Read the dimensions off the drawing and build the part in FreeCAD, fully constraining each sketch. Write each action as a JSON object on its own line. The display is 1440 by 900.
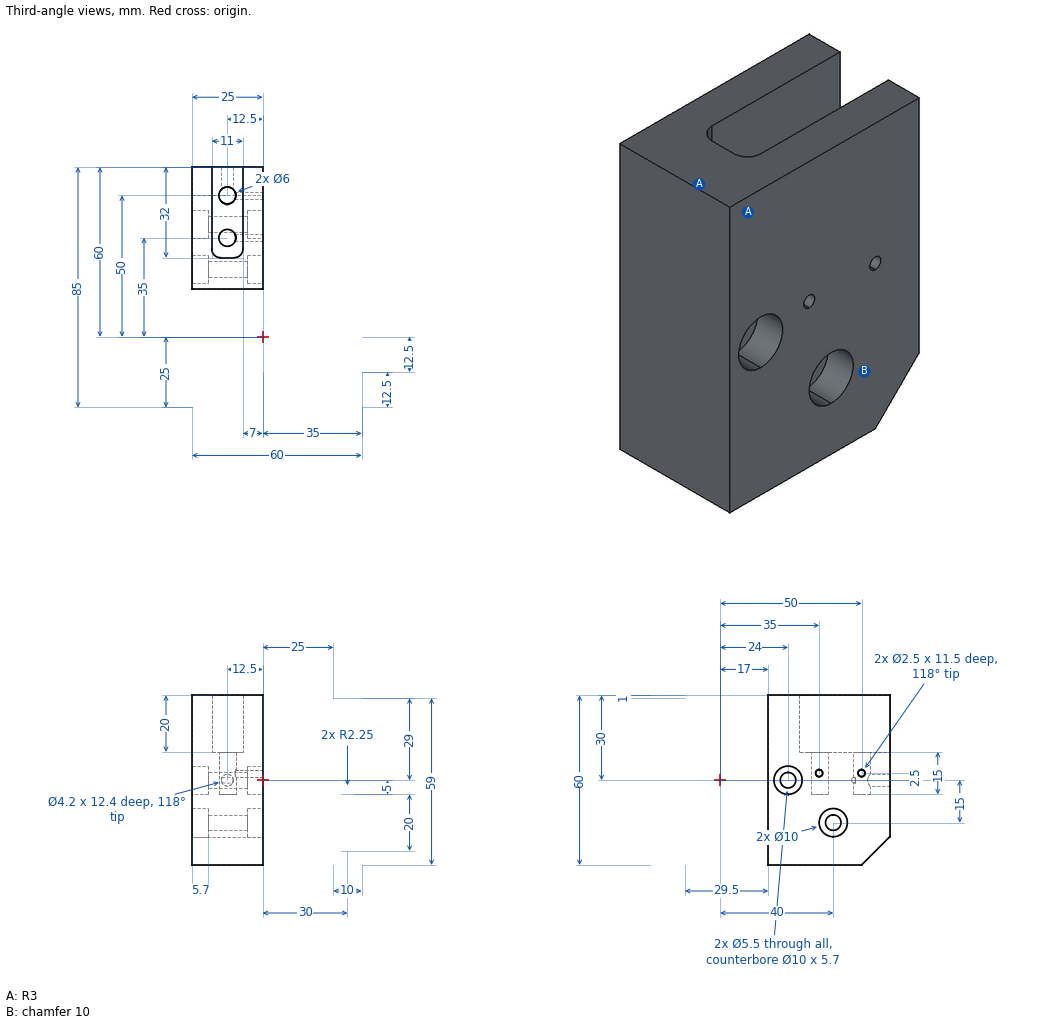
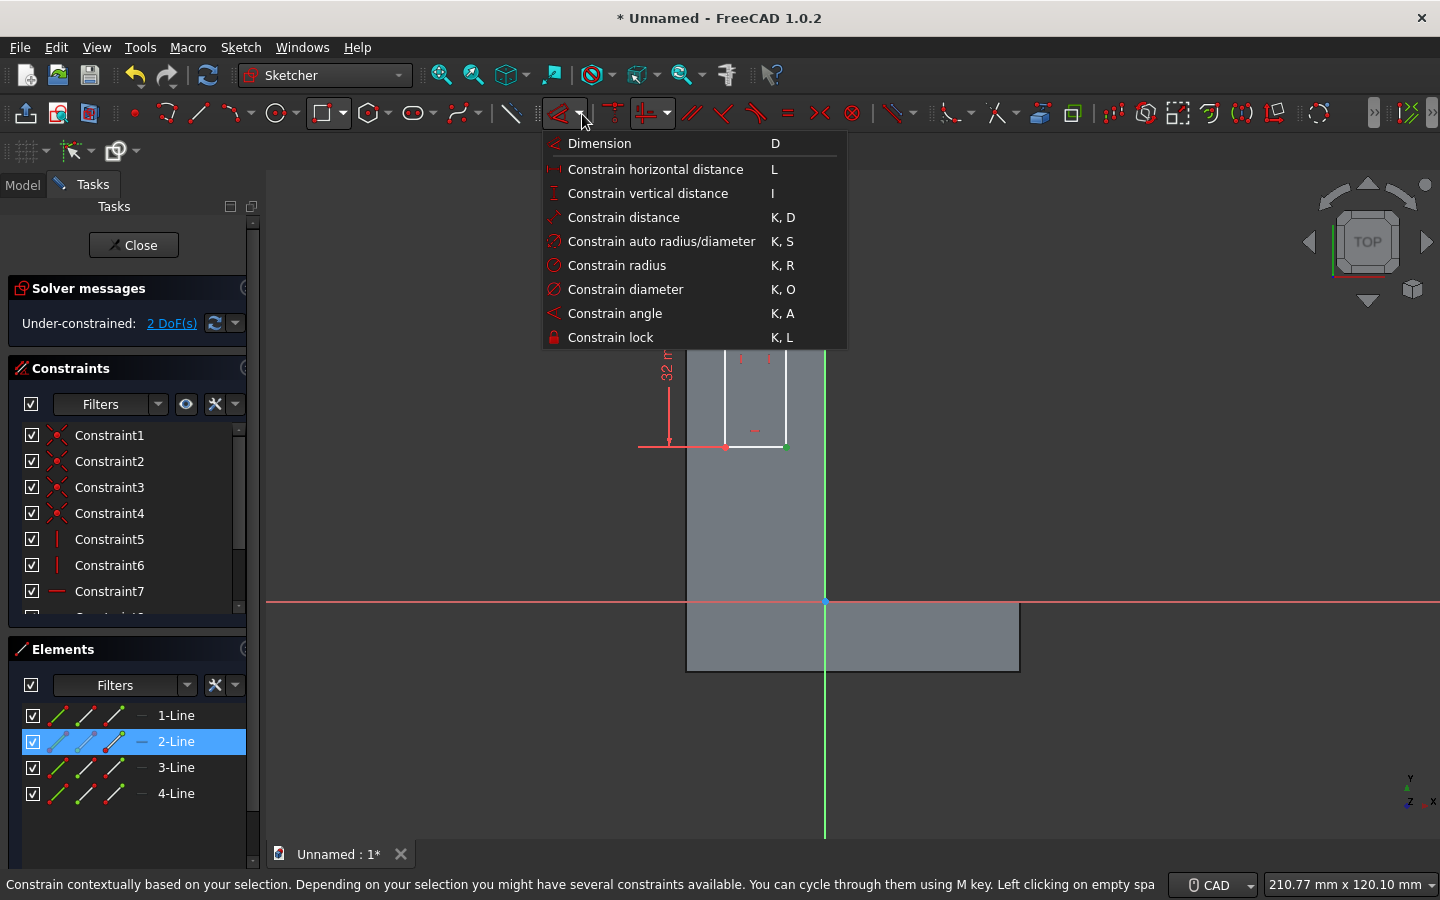
{"action": "left_click", "coordinate": [695, 169]}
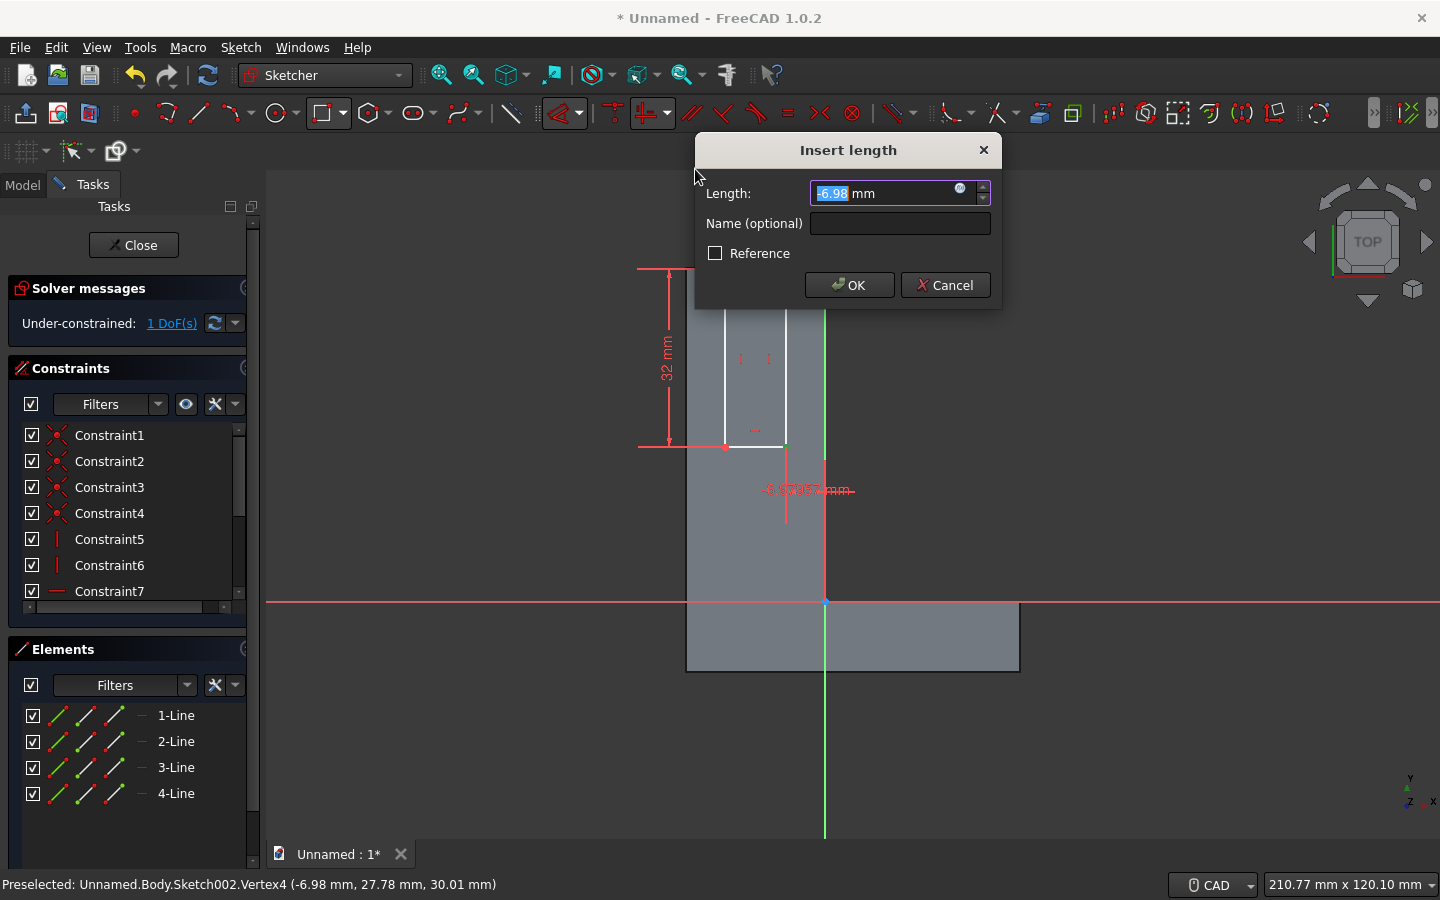
{"action": "type", "text": "-7"}
{"action": "key", "text": "Return"}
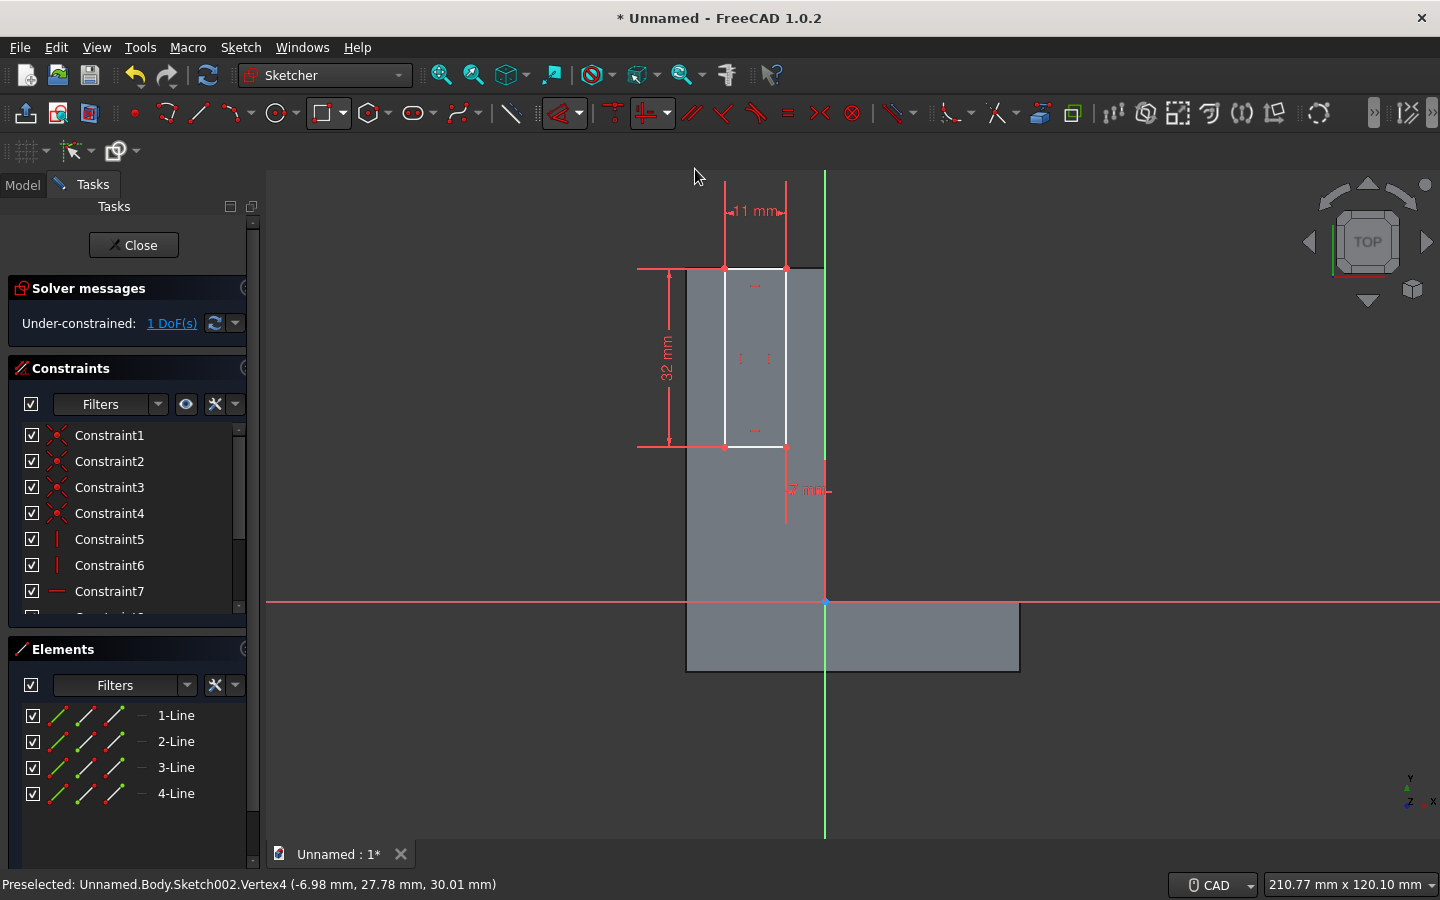
{"action": "left_click", "coordinate": [725, 269]}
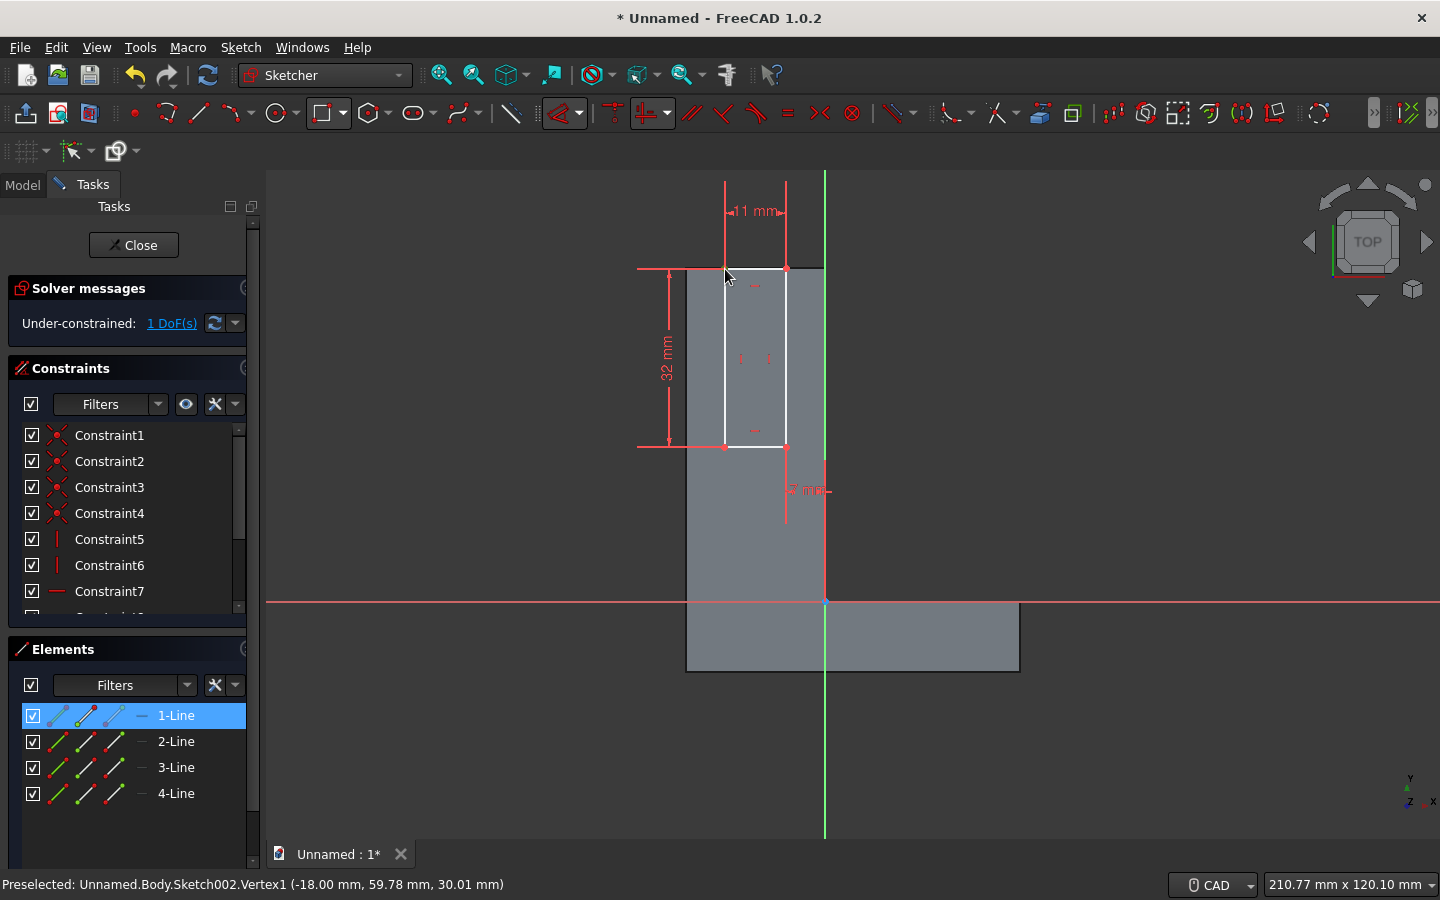
{"action": "left_click", "coordinate": [582, 114]}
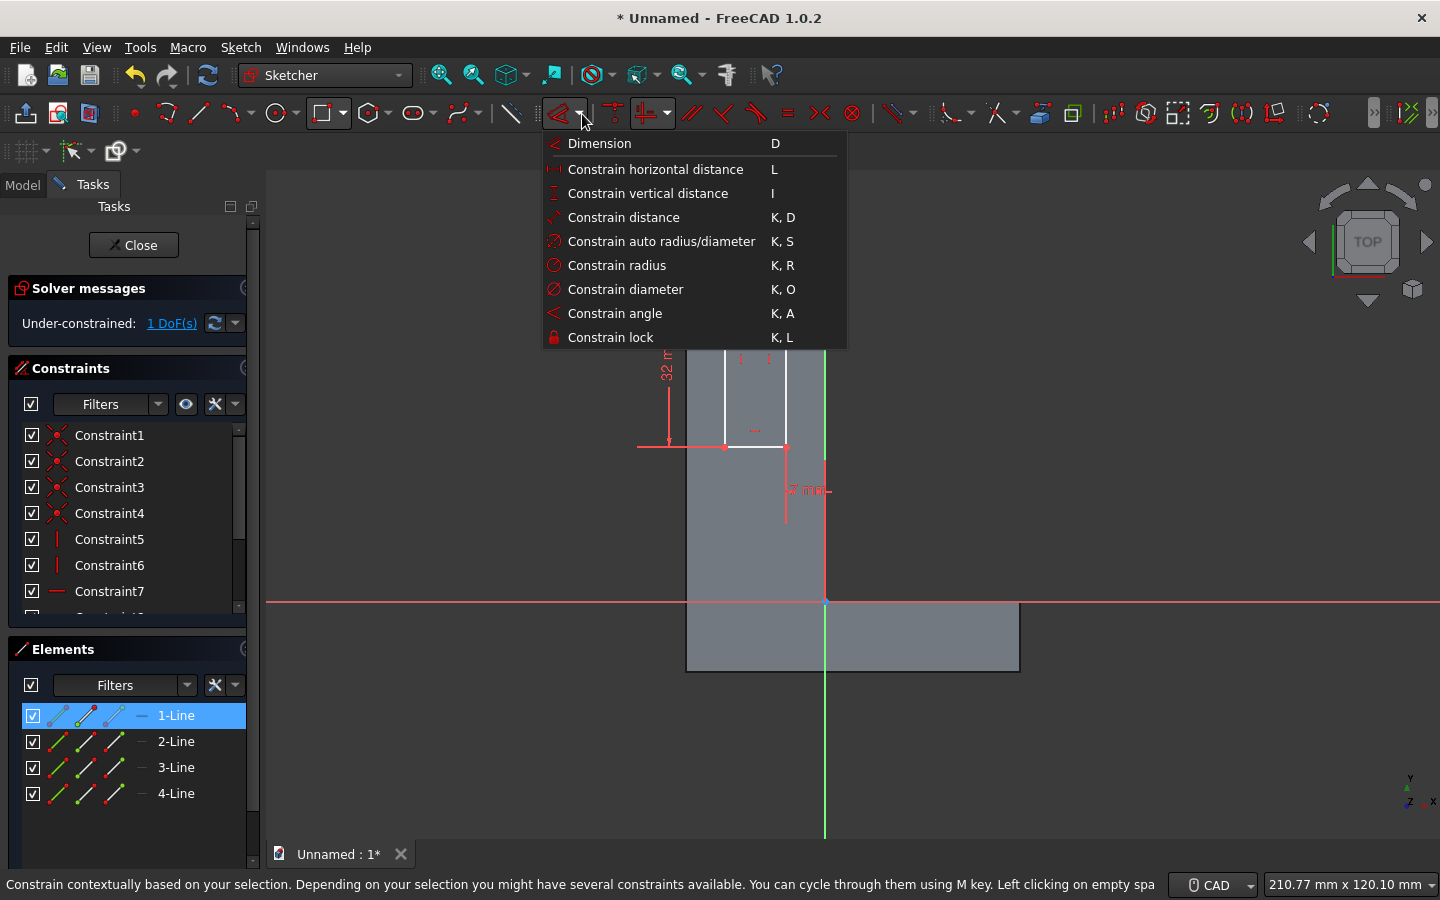
{"action": "left_click", "coordinate": [695, 193]}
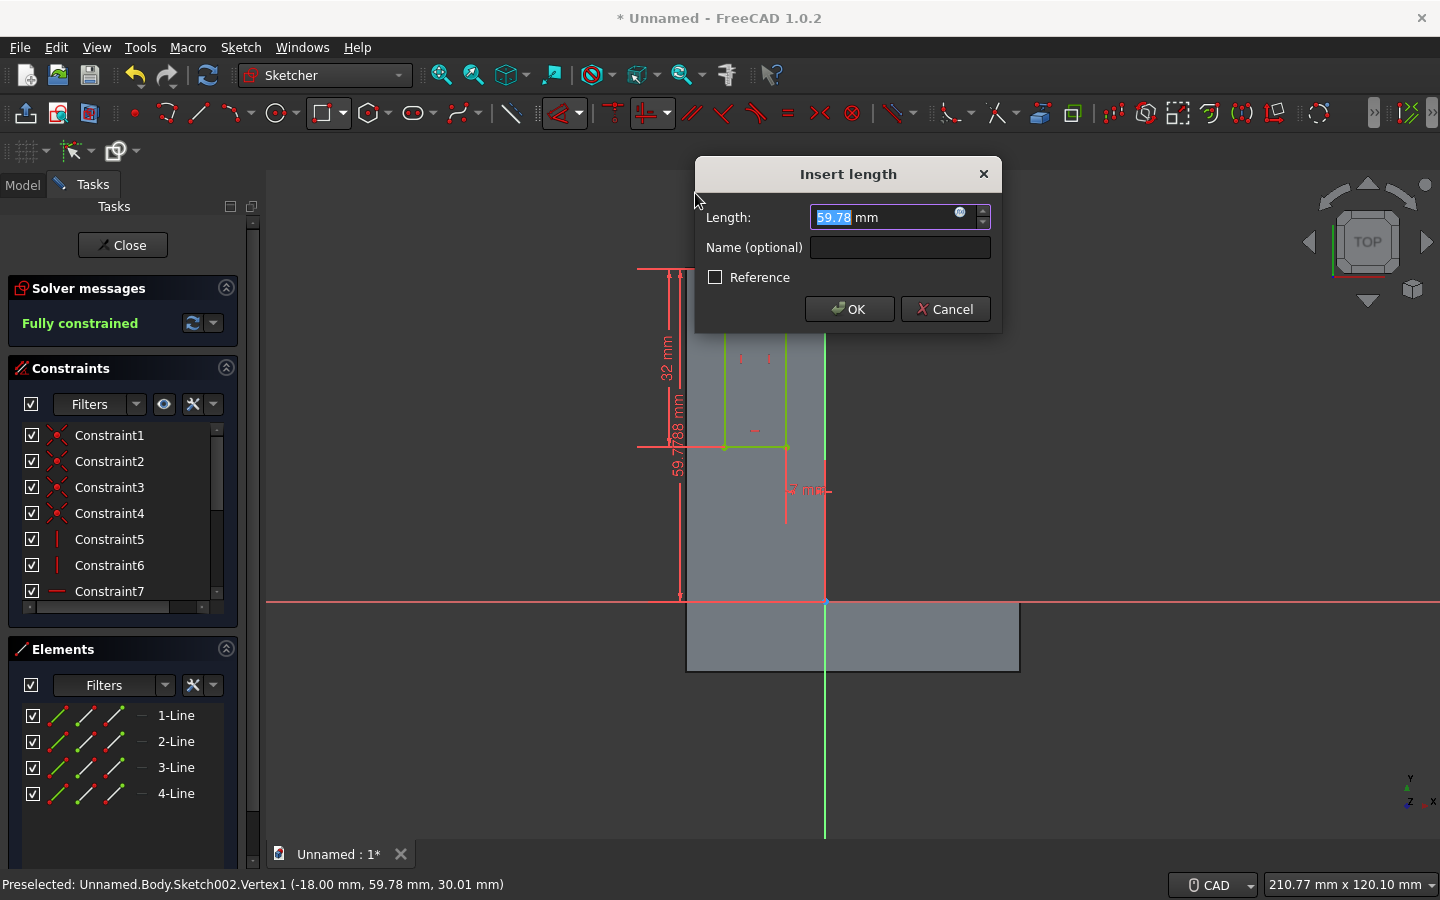
{"action": "type", "text": "60"}
{"action": "key", "text": "Return"}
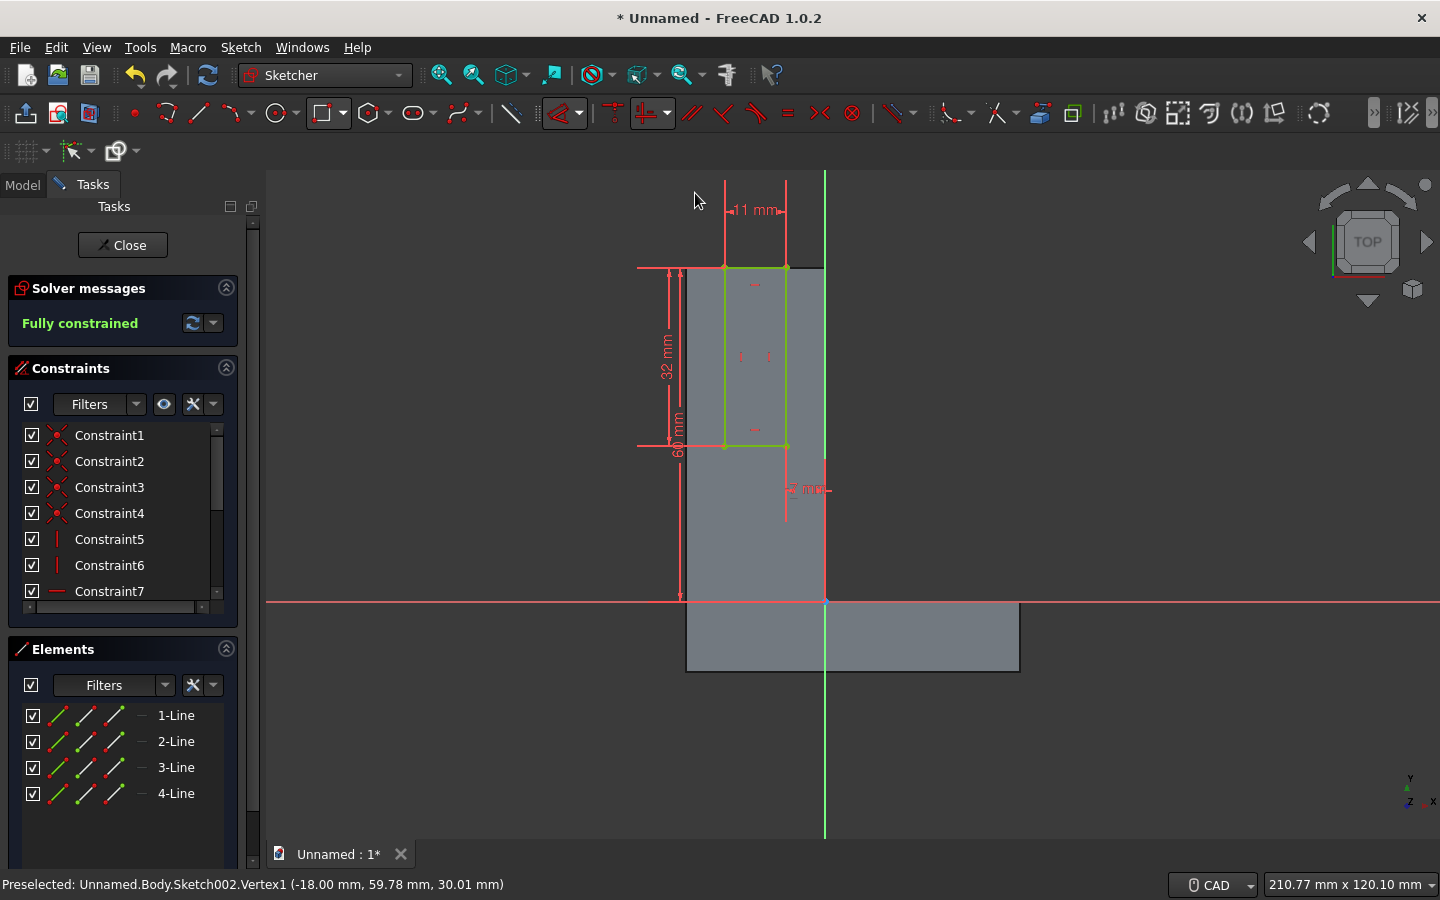
{"action": "left_click", "coordinate": [123, 245]}